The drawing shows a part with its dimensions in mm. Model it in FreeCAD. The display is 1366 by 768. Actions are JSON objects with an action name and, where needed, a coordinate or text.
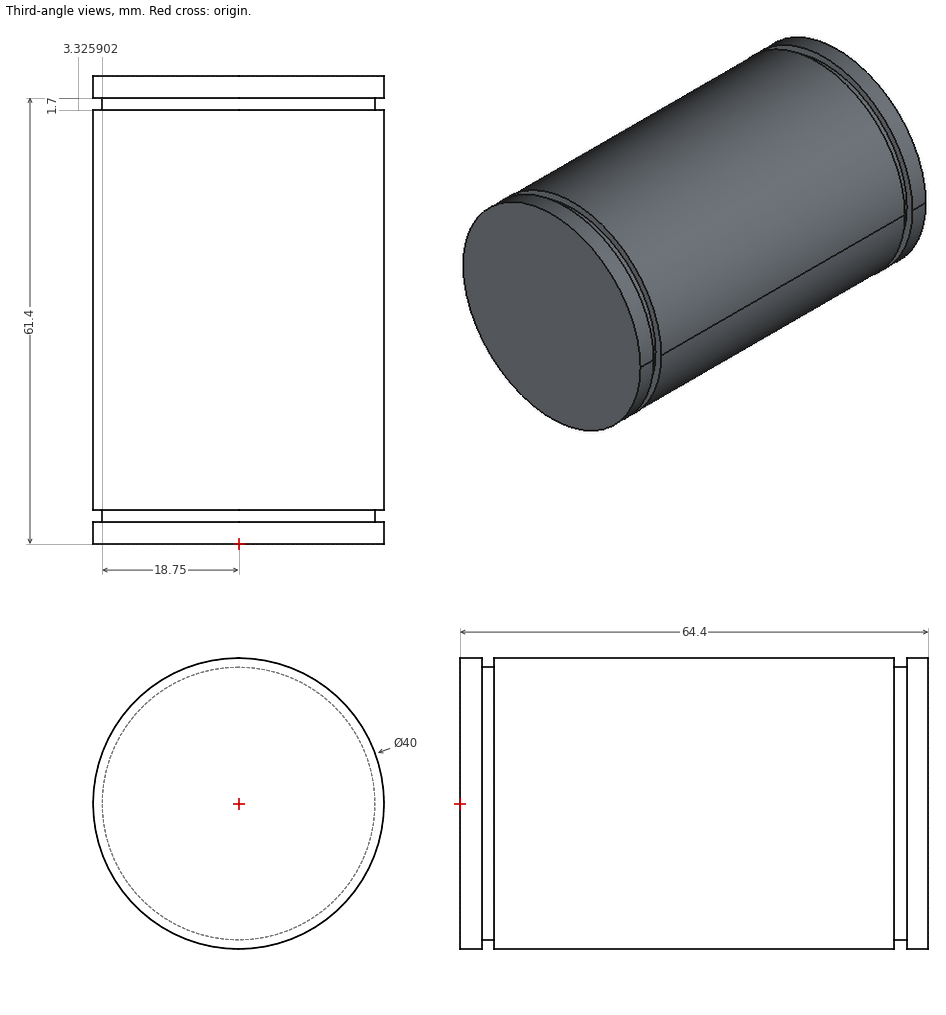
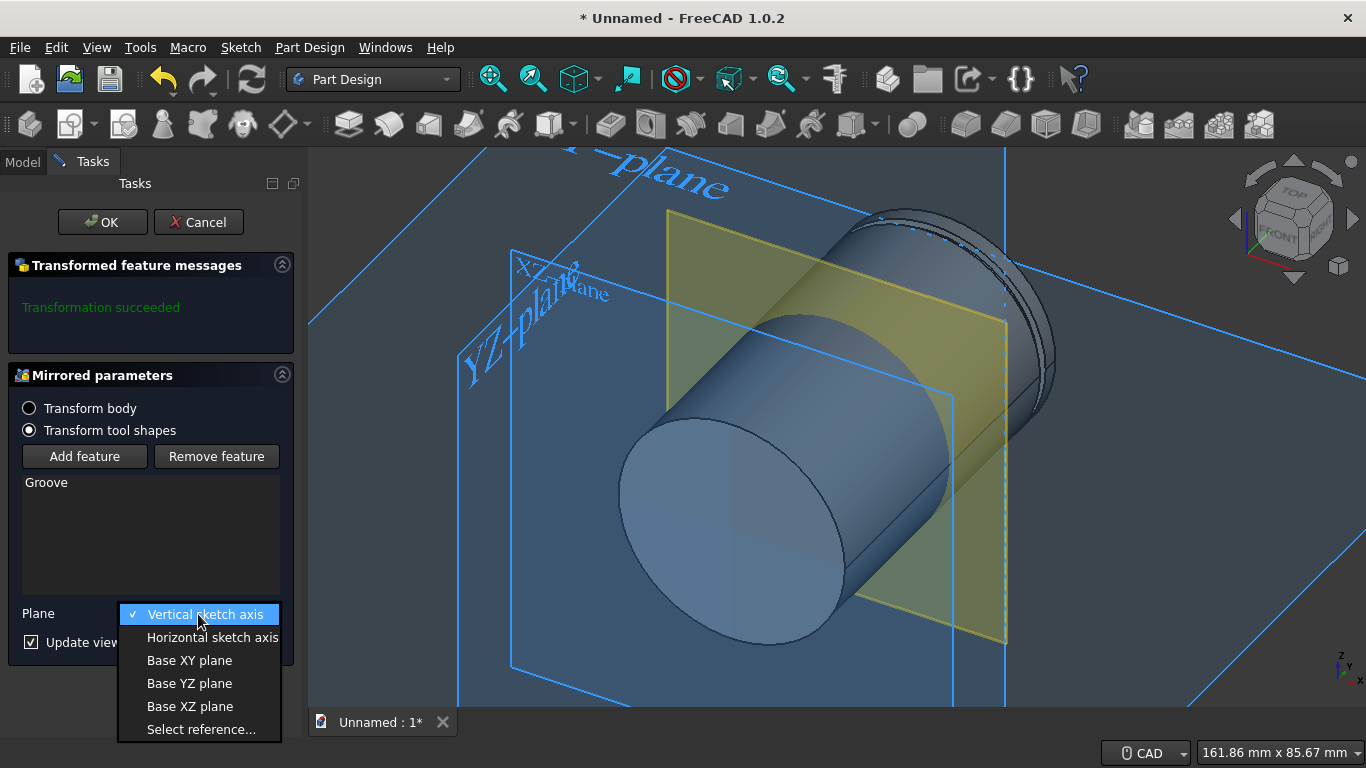
{"action": "left_click", "coordinate": [198, 730]}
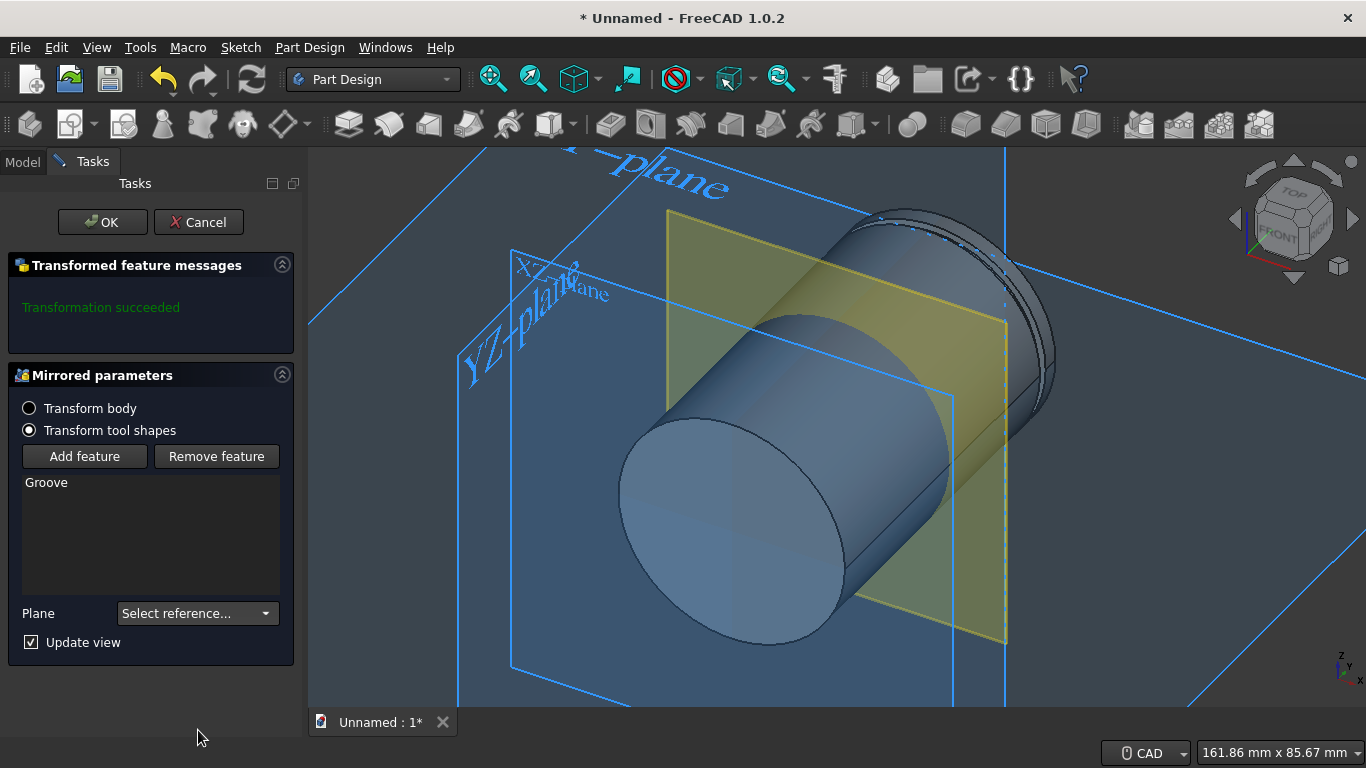
{"action": "left_click", "coordinate": [23, 161]}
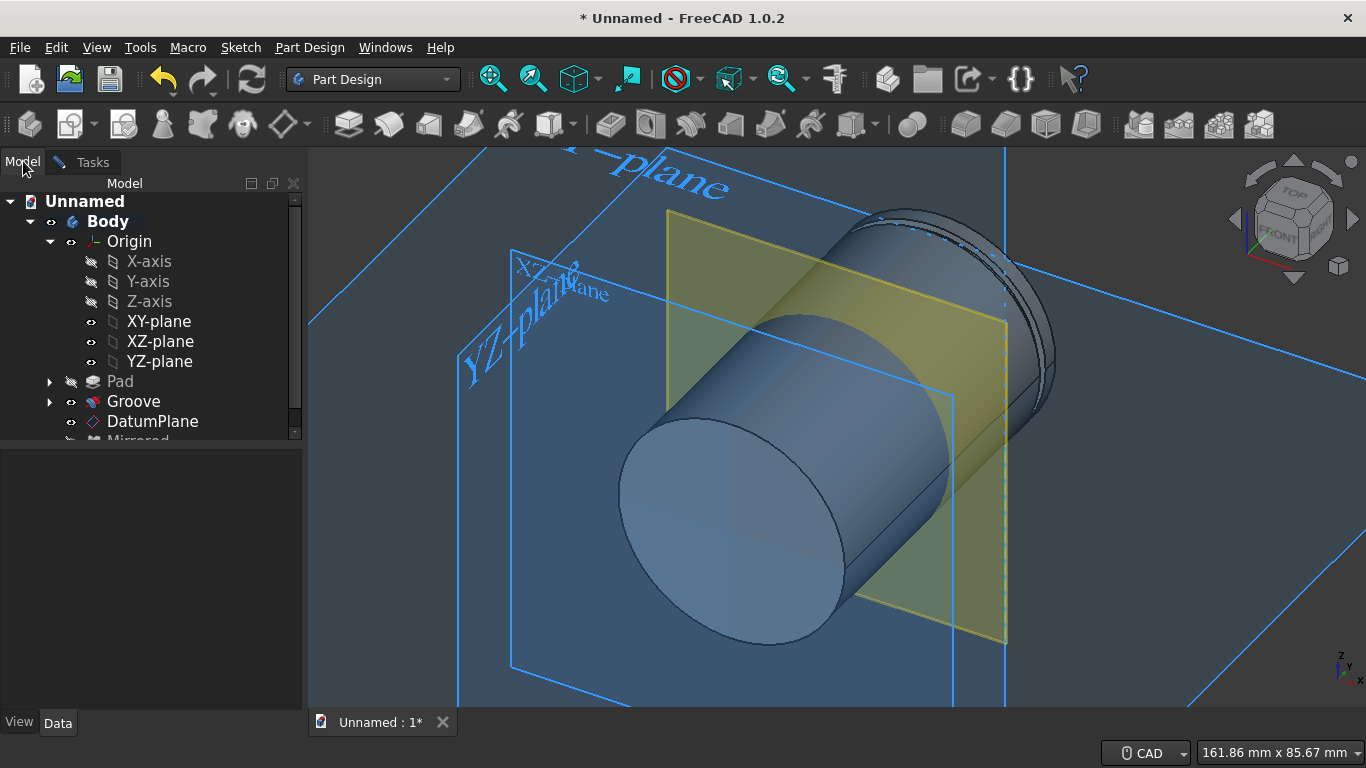
{"action": "left_click", "coordinate": [116, 422]}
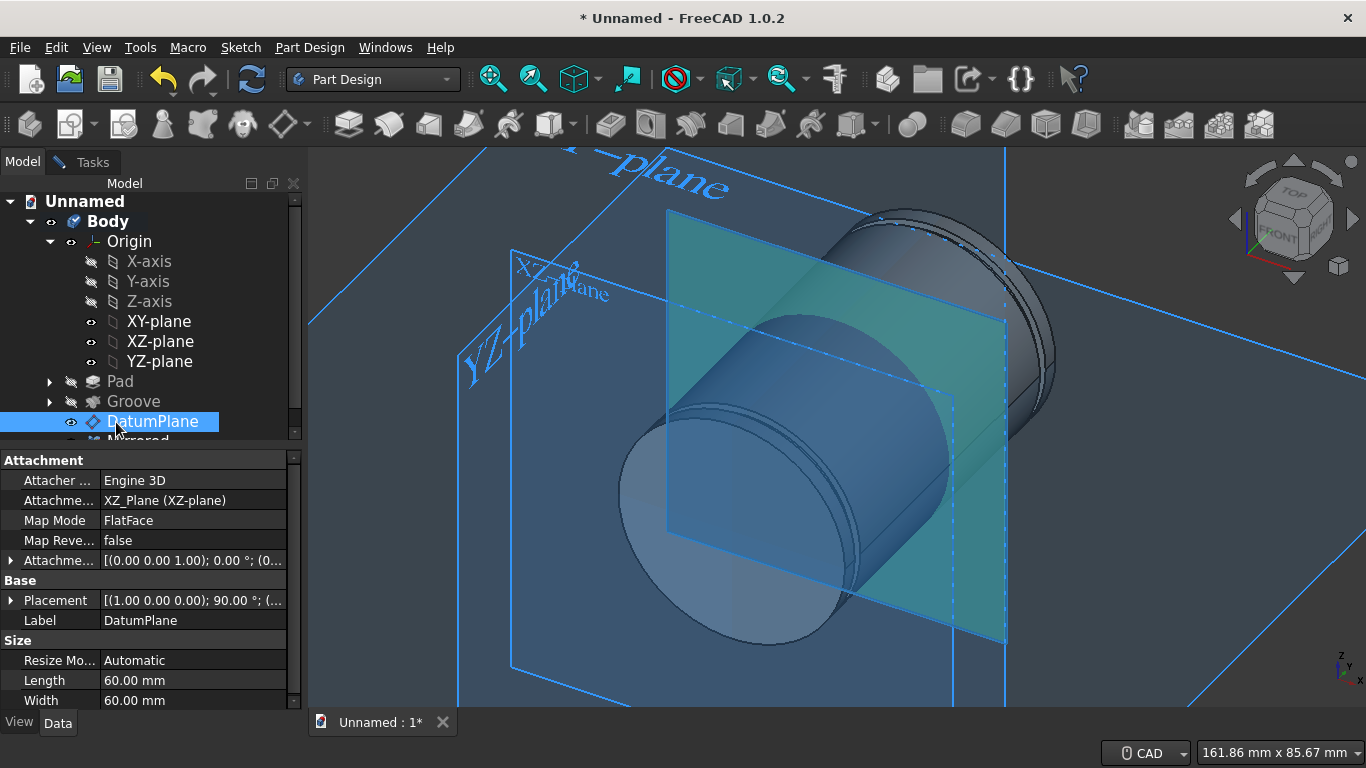
{"action": "left_click", "coordinate": [84, 161]}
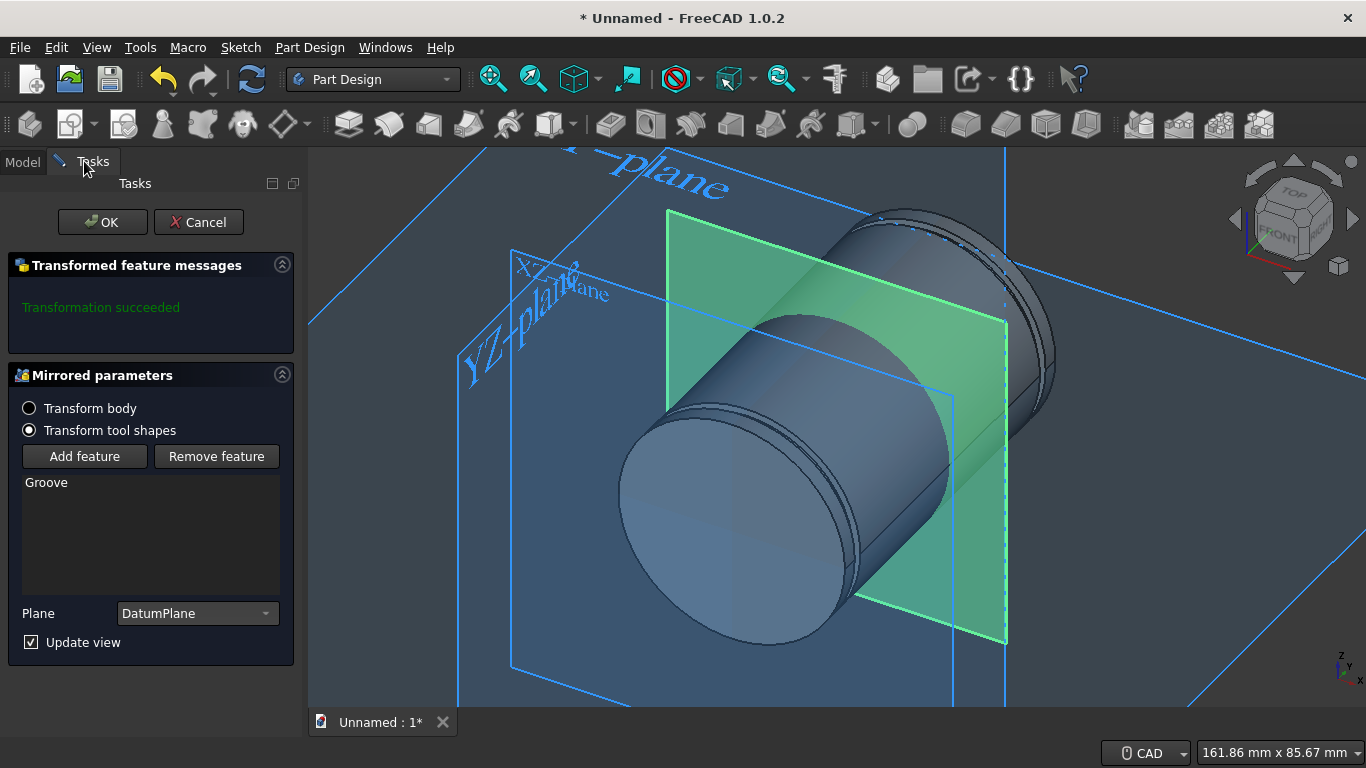
{"action": "left_click", "coordinate": [103, 222]}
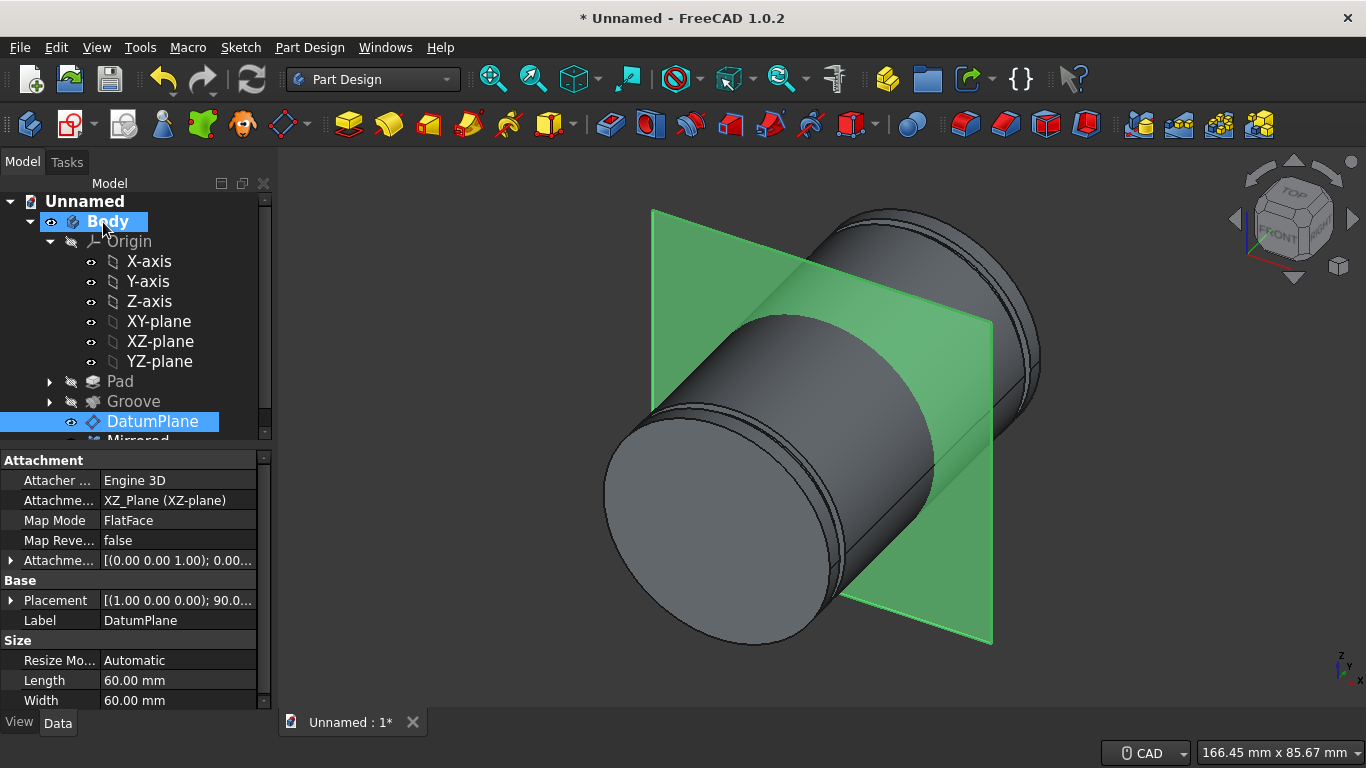
{"action": "left_click", "coordinate": [116, 422]}
{"action": "key", "text": "space"}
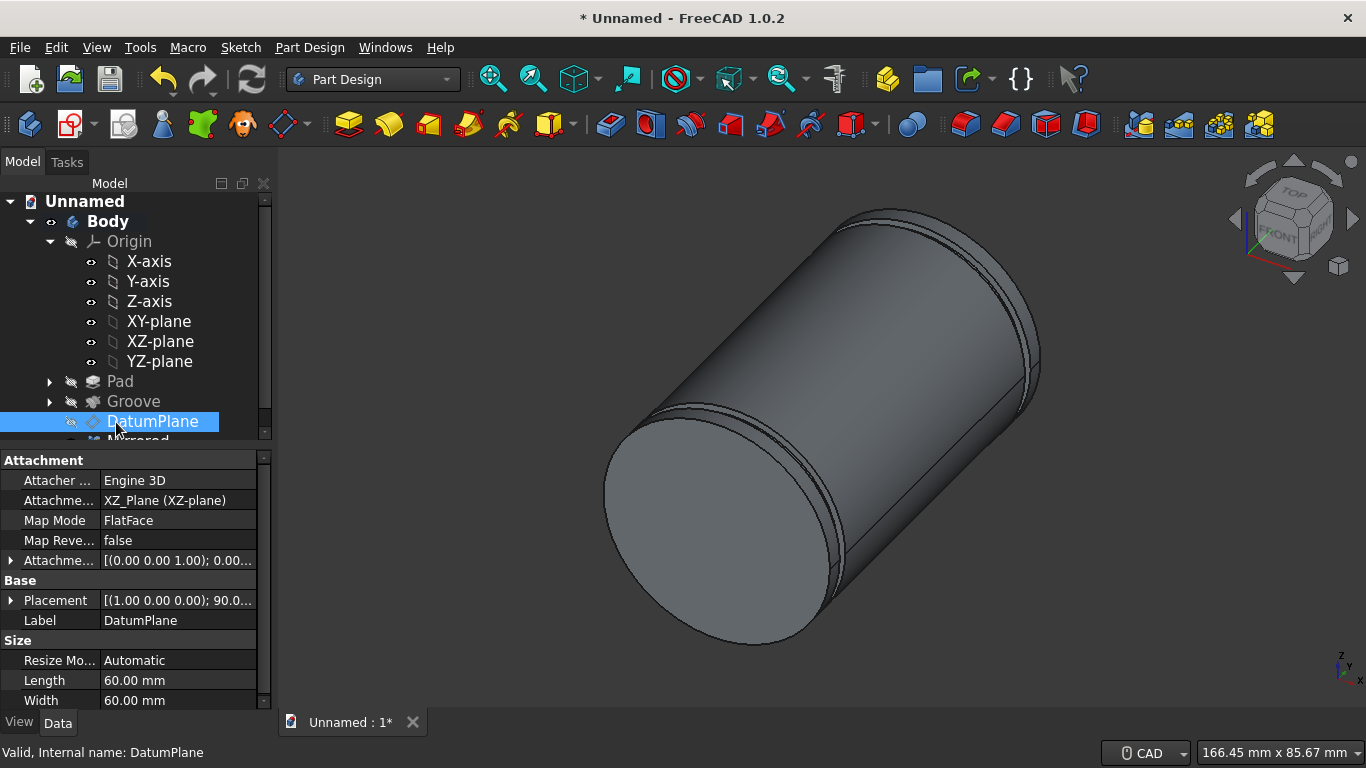
{"action": "key", "text": "0"}